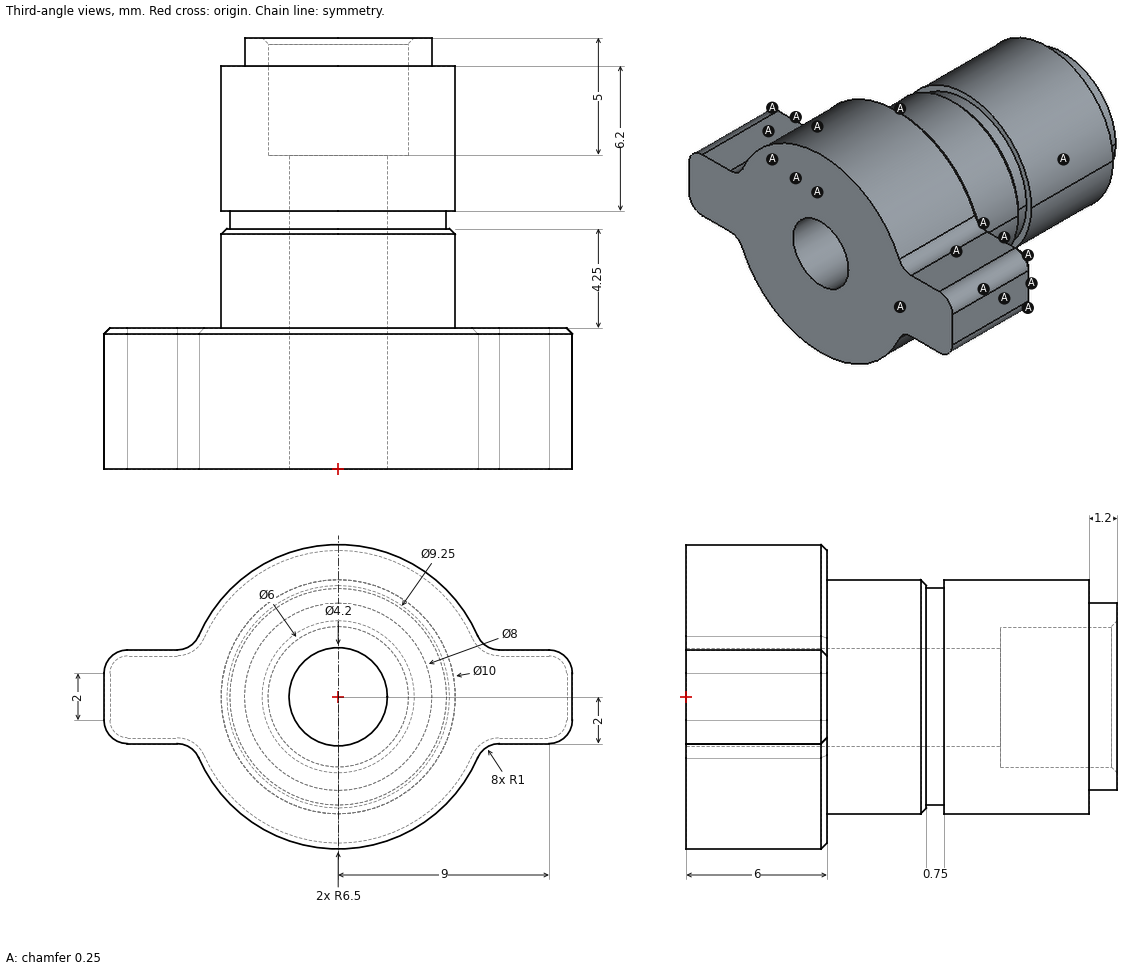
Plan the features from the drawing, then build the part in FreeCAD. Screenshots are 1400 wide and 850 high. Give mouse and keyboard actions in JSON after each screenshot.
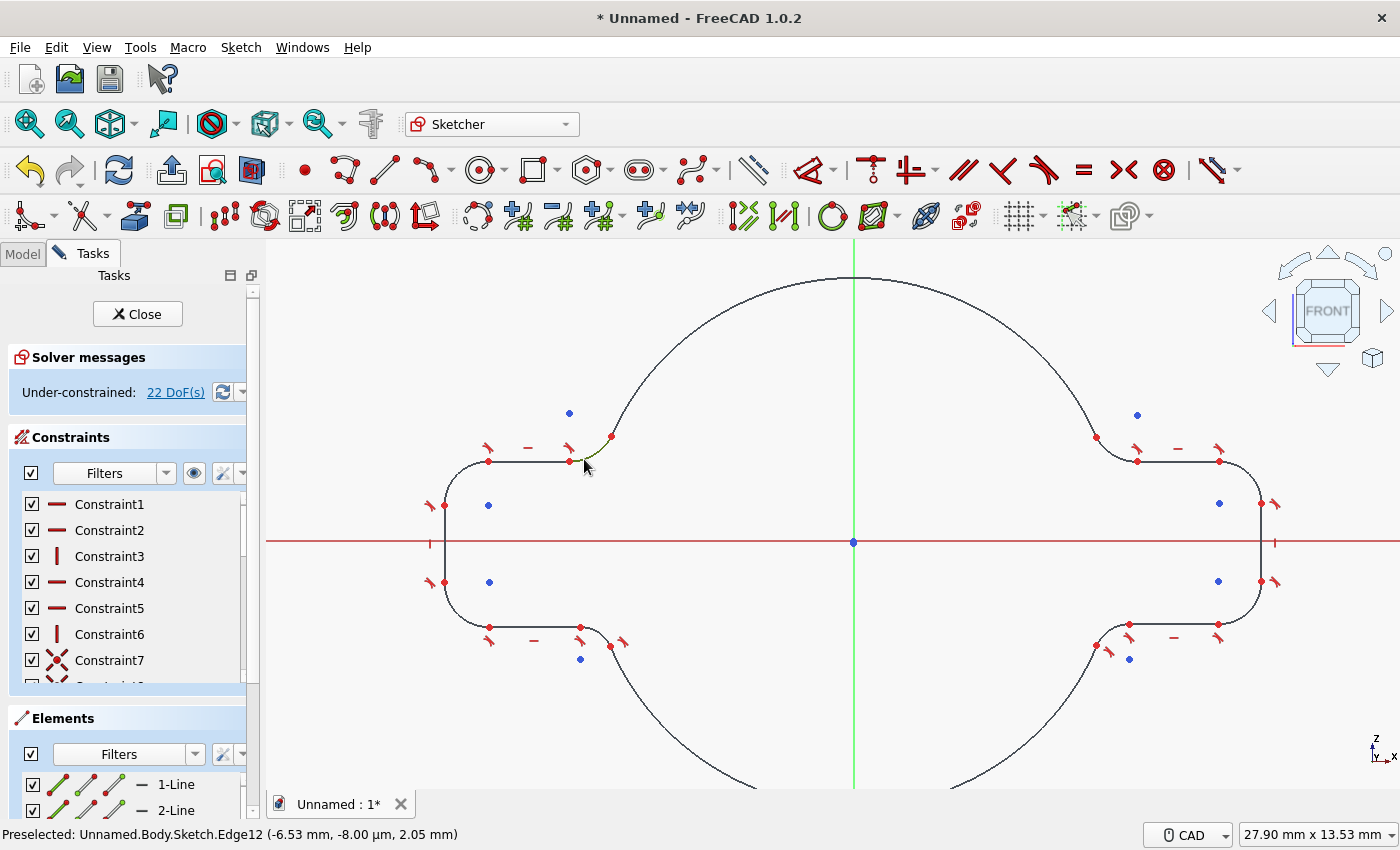
{"action": "left_click", "coordinate": [972, 306]}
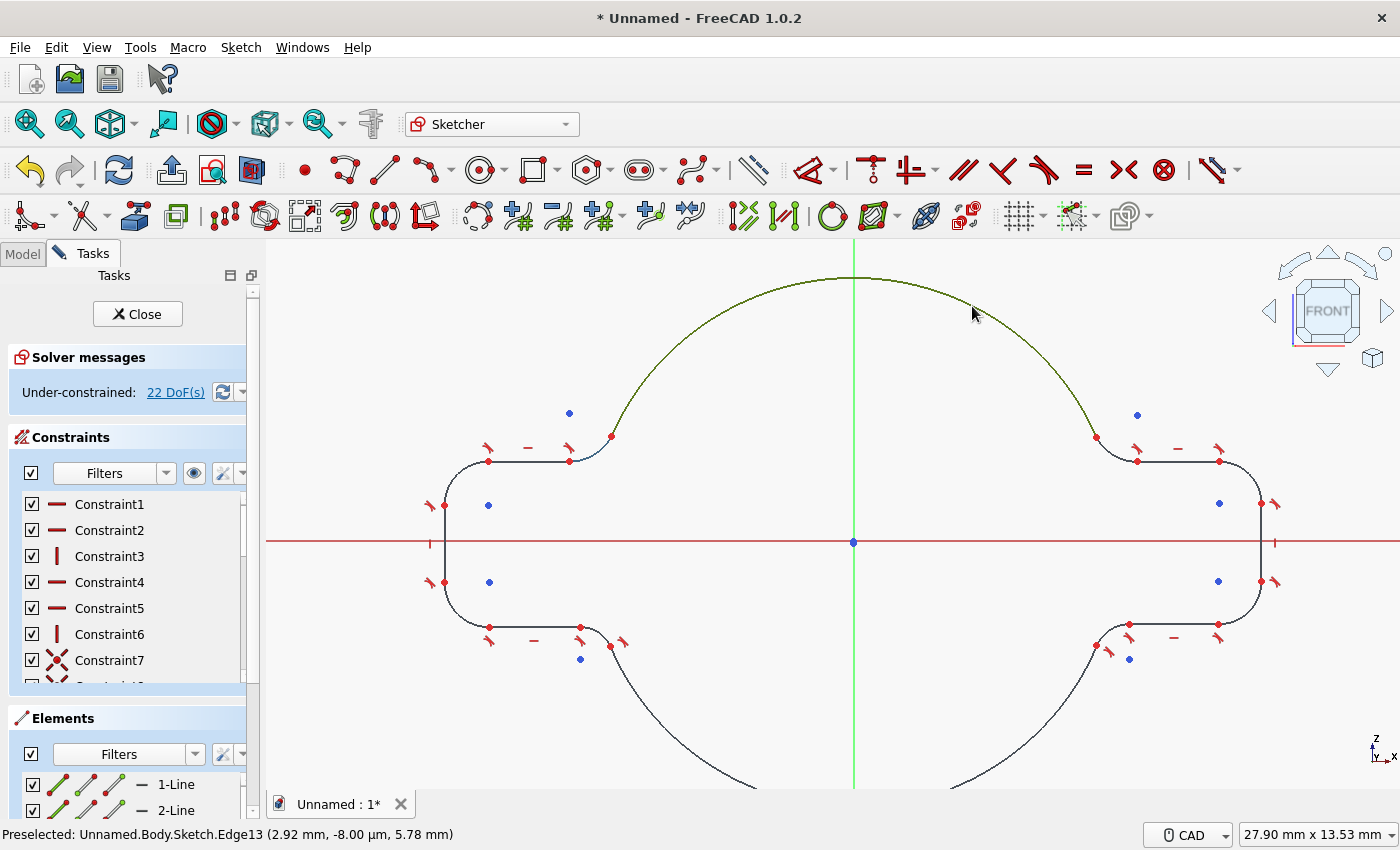
{"action": "left_click", "coordinate": [1044, 170]}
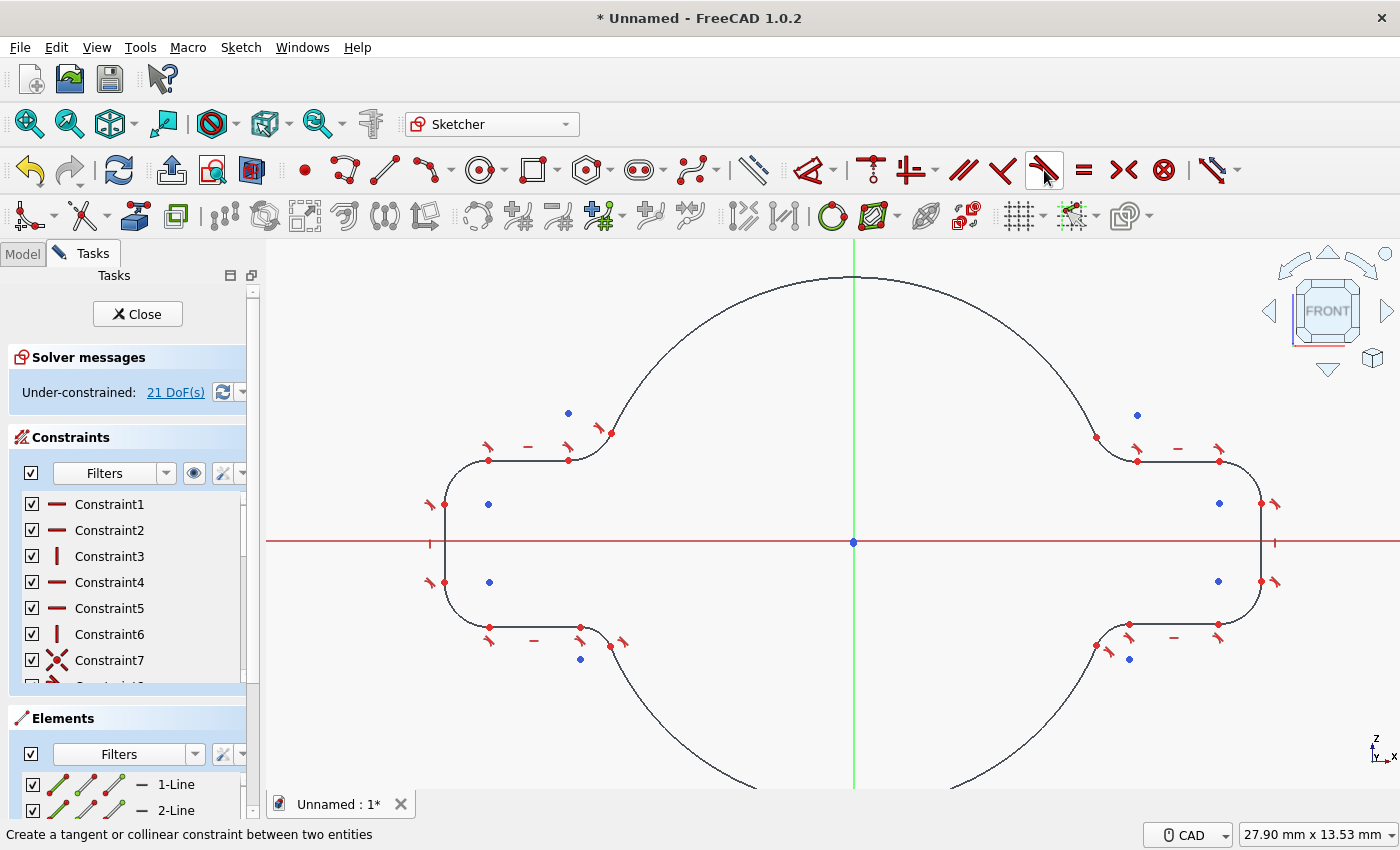
{"action": "left_click", "coordinate": [973, 306]}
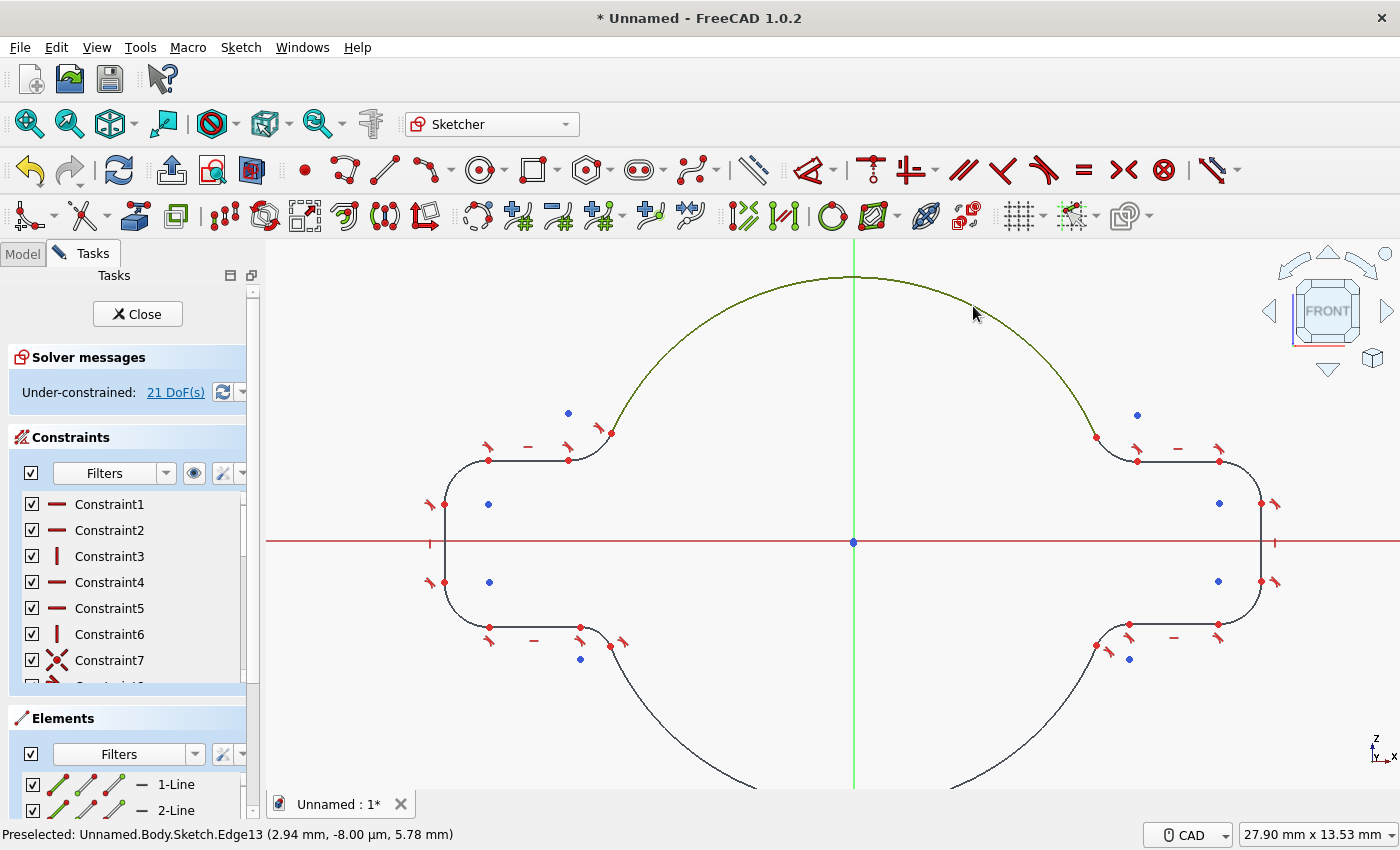
{"action": "left_click", "coordinate": [1106, 449]}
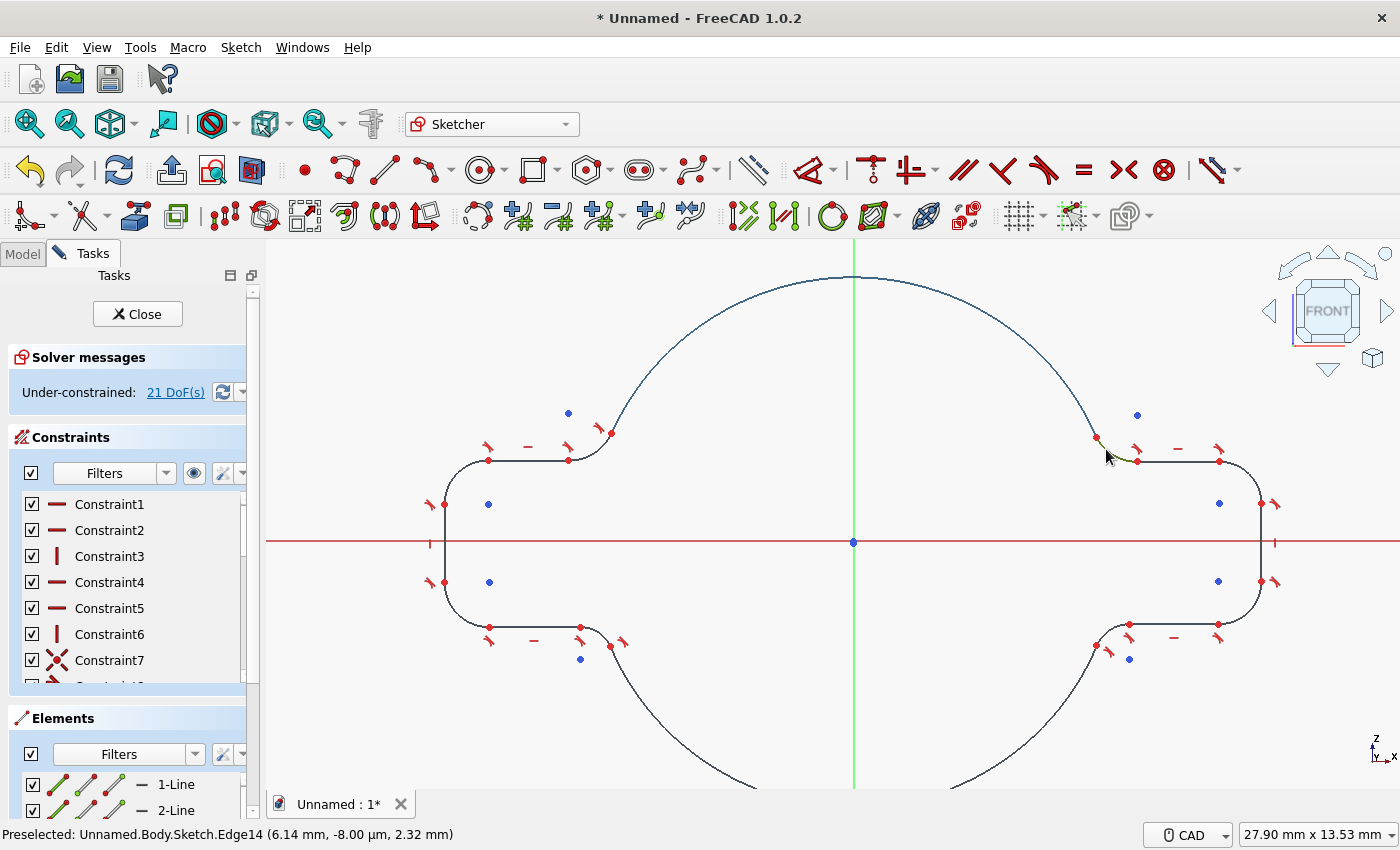
{"action": "left_click", "coordinate": [1044, 170]}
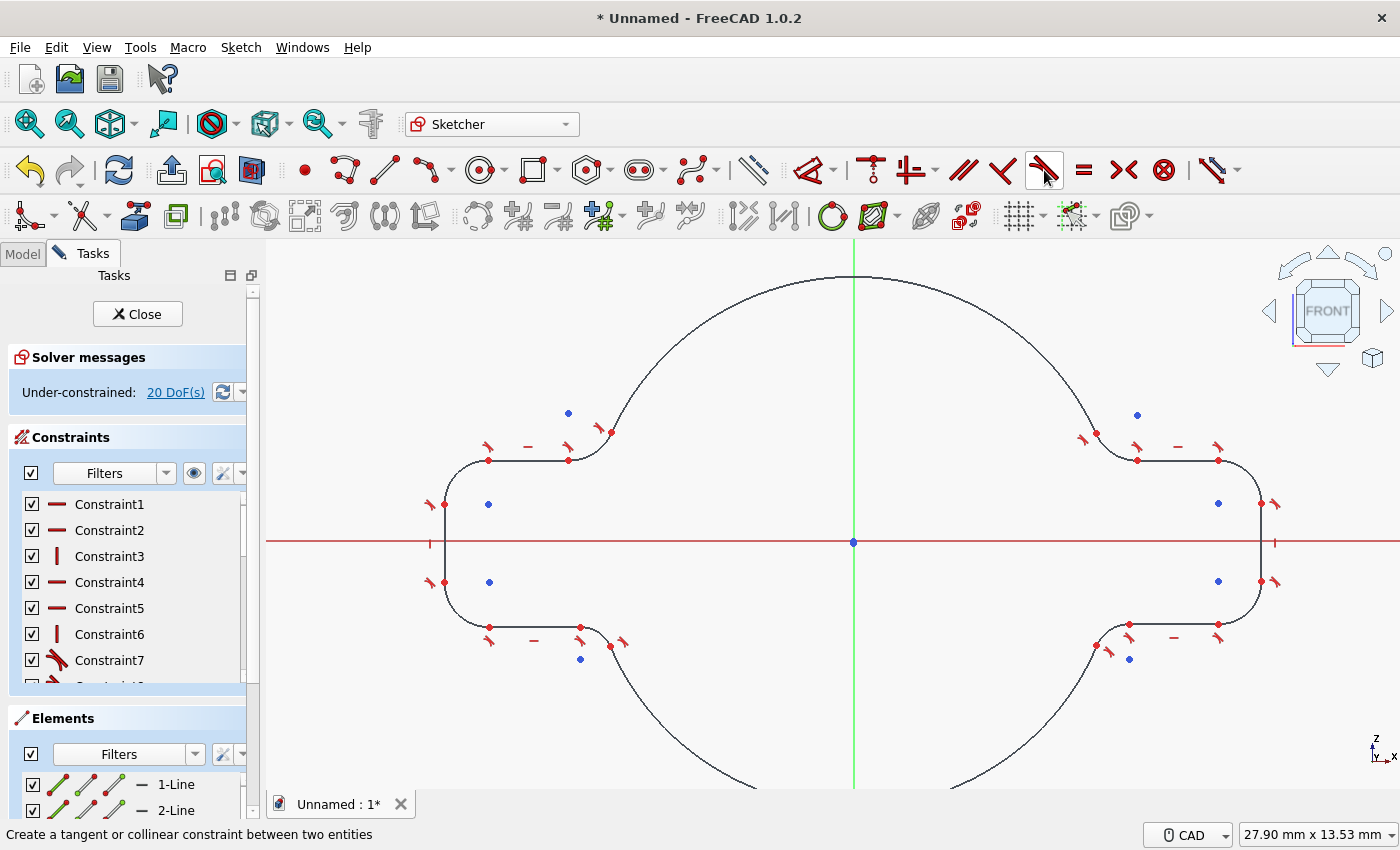
{"action": "left_click", "coordinate": [683, 745]}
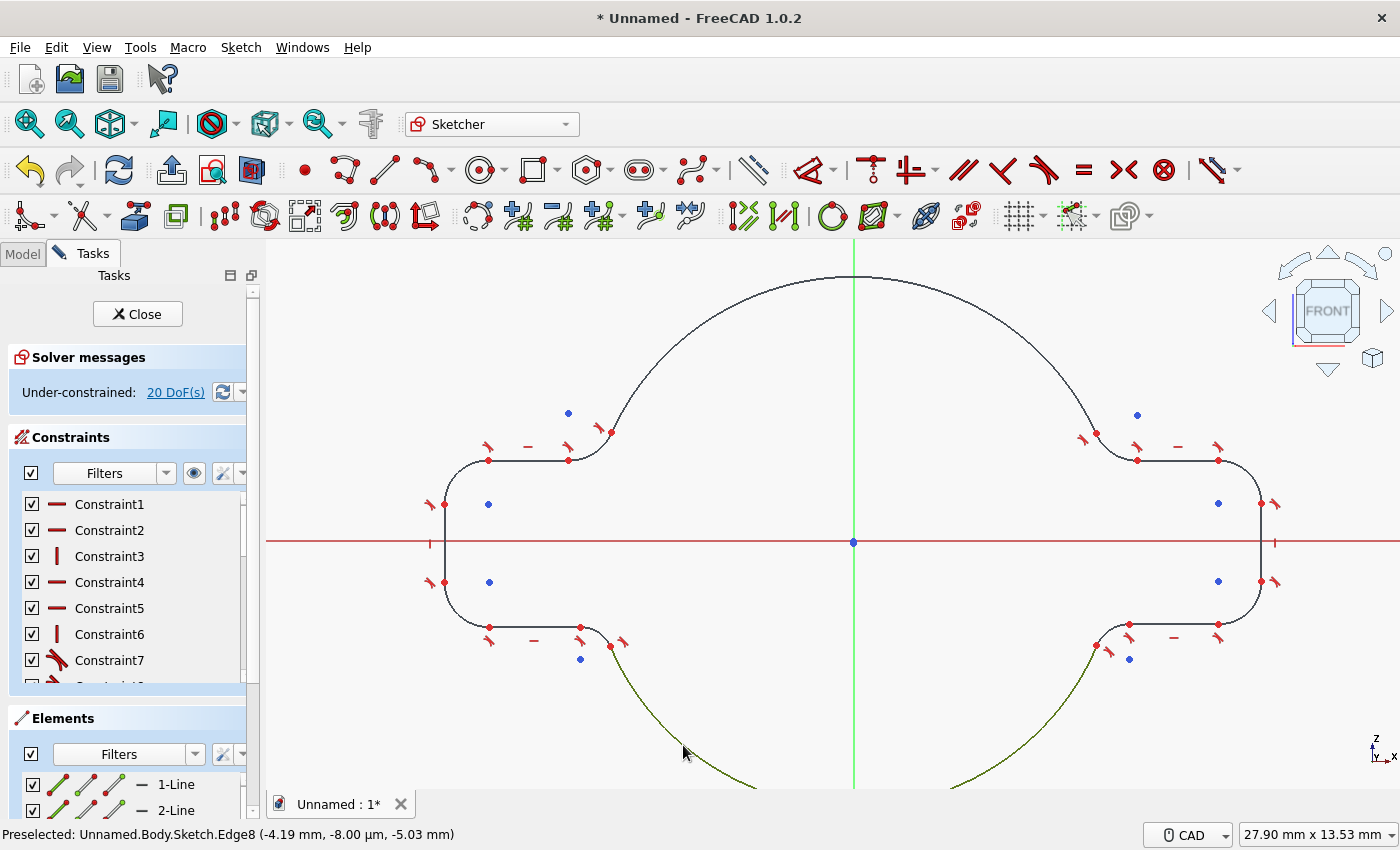
{"action": "left_click", "coordinate": [972, 305]}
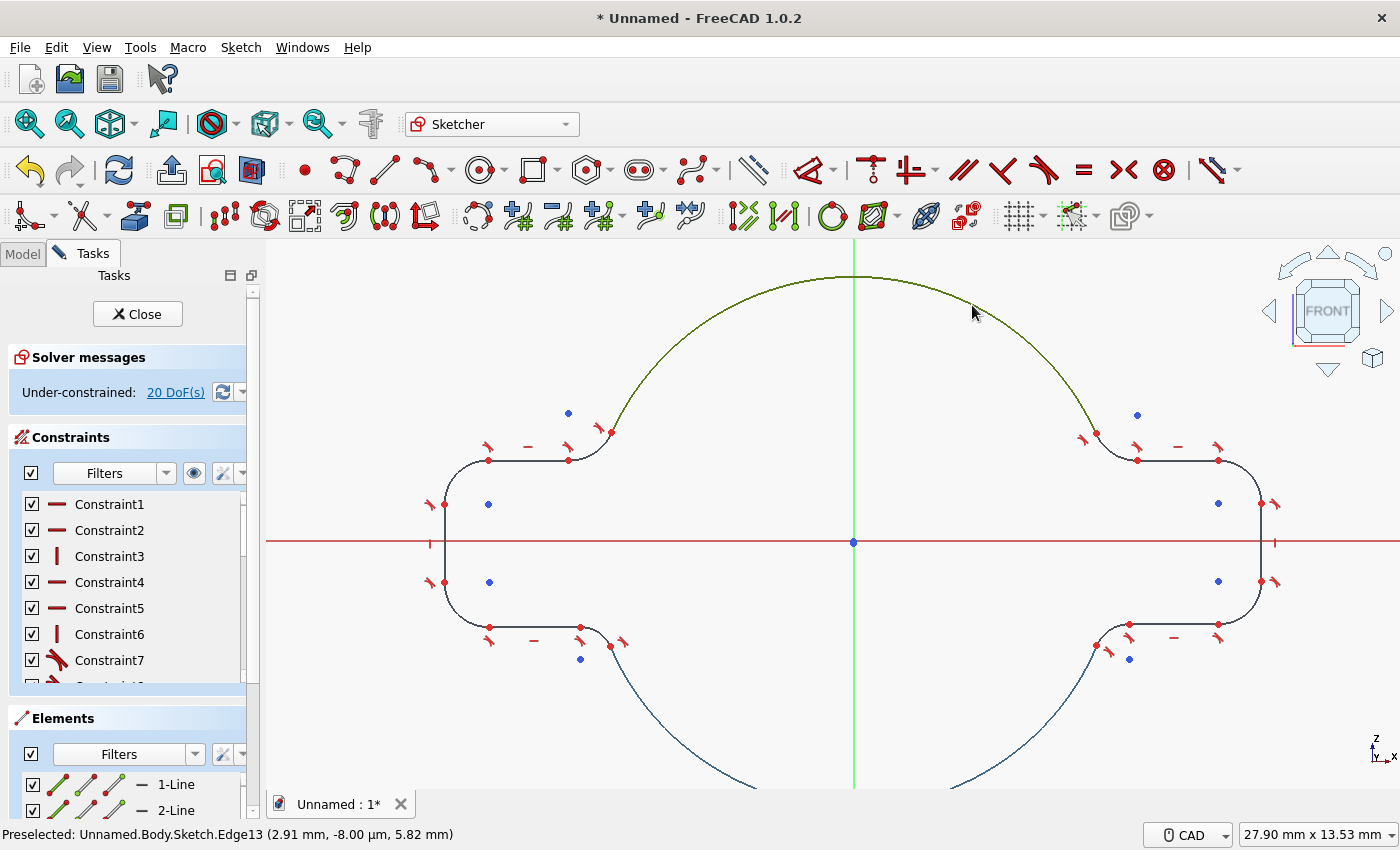
{"action": "left_click", "coordinate": [872, 170]}